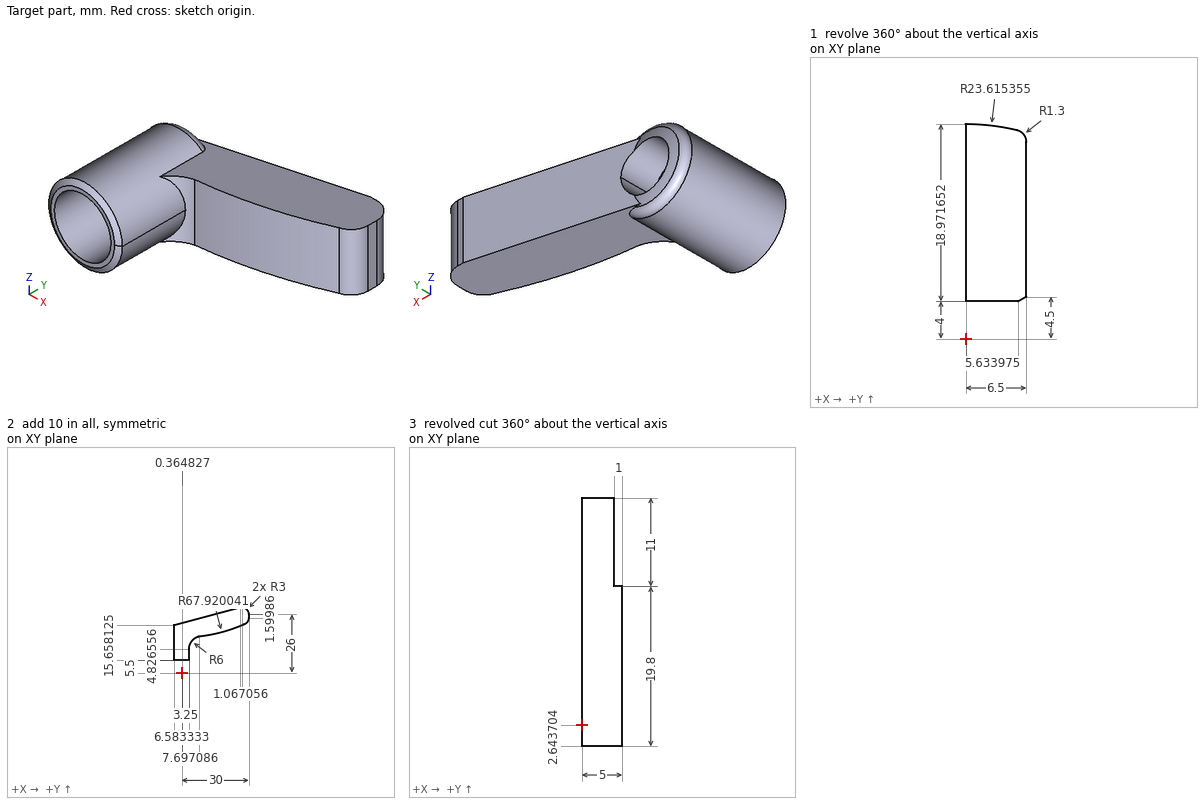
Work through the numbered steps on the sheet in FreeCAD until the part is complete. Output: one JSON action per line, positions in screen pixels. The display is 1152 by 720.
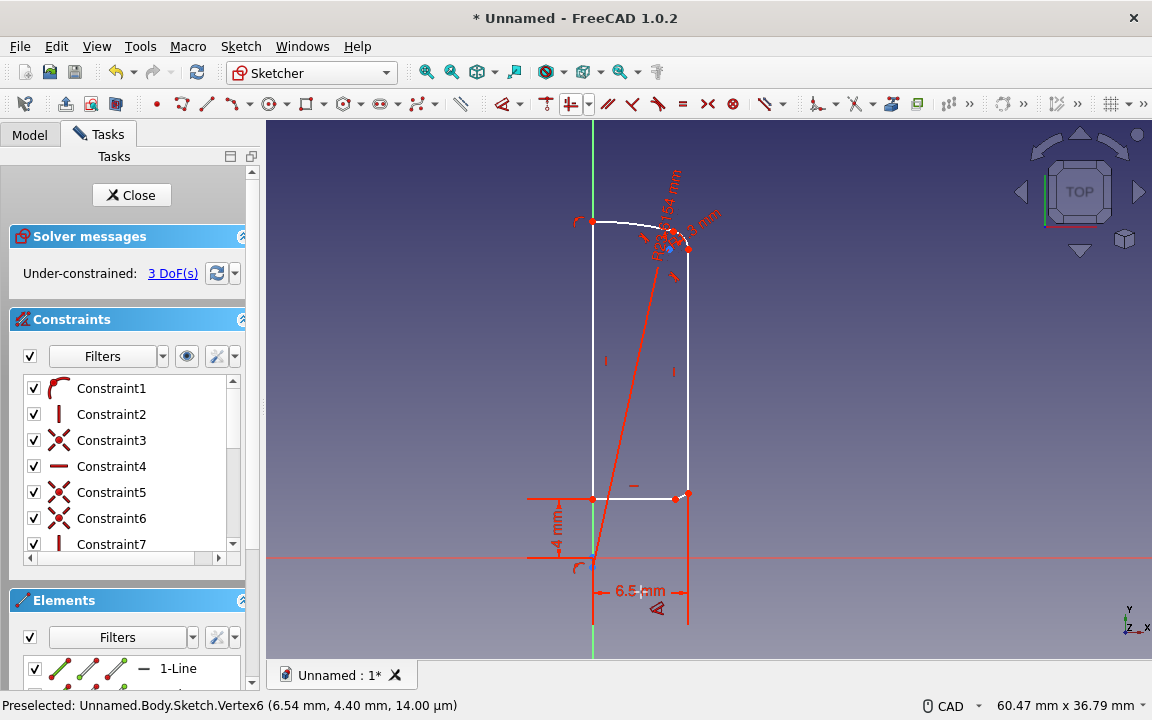
{"action": "left_click", "coordinate": [688, 494]}
{"action": "left_click", "coordinate": [722, 526]}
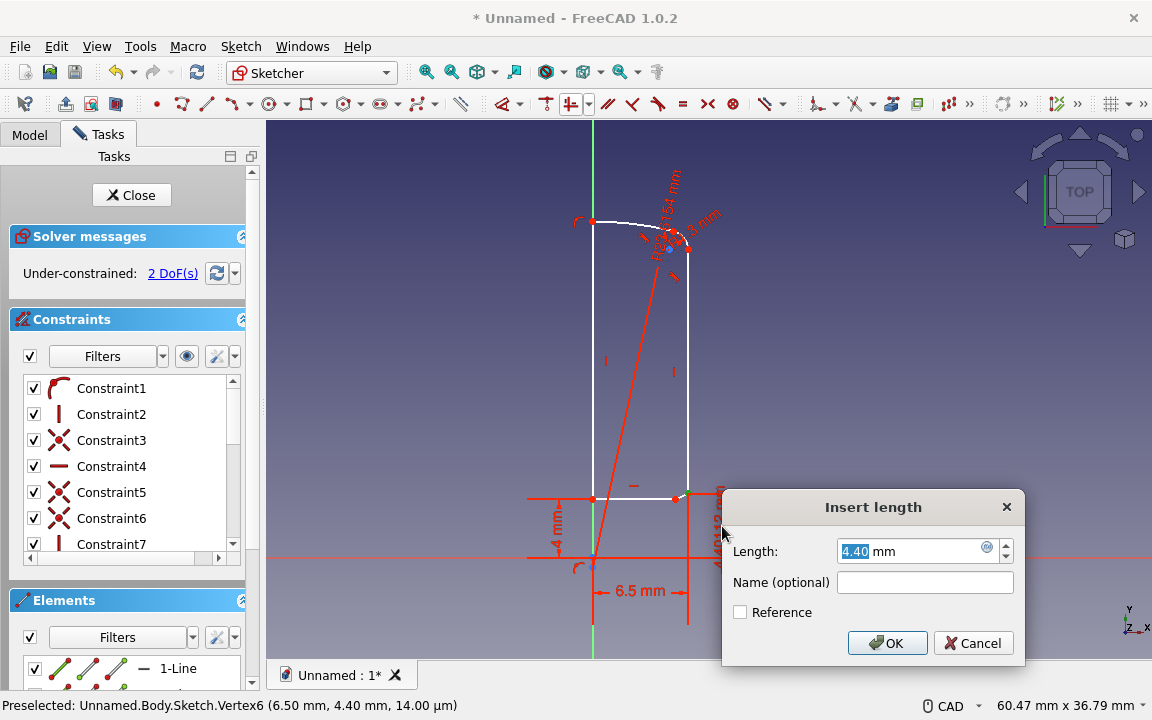
{"action": "type", "text": "4.5"}
{"action": "key", "text": "Return"}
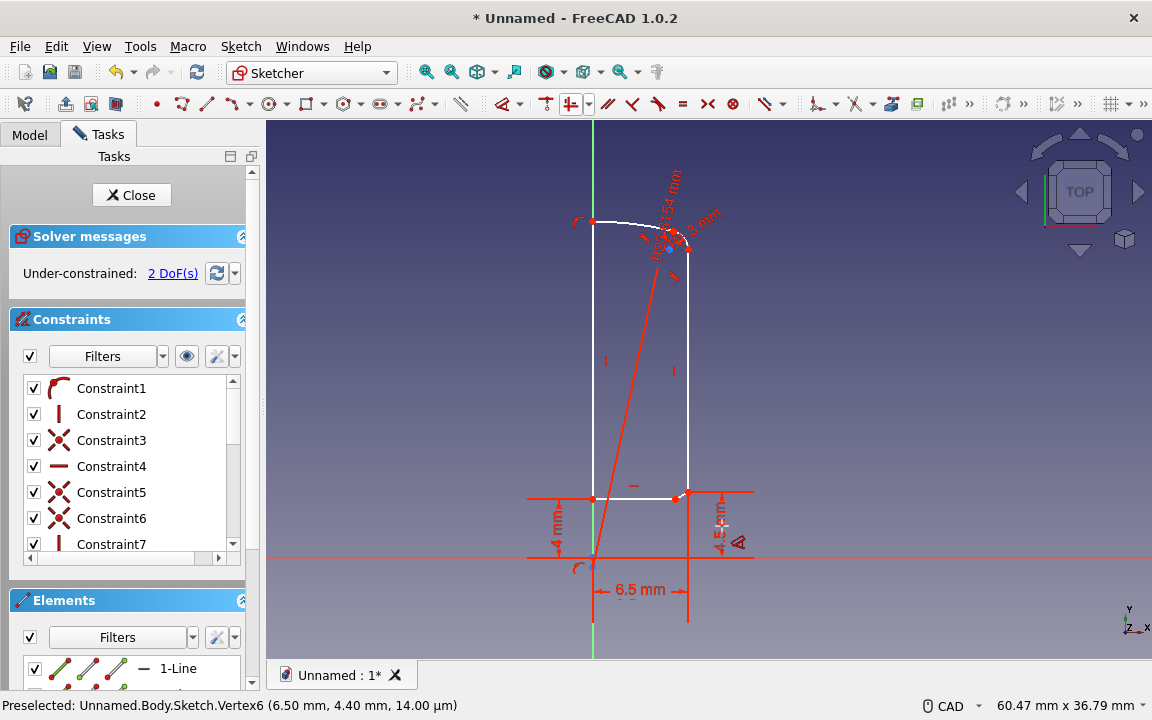
{"action": "left_click", "coordinate": [618, 499]}
{"action": "left_click", "coordinate": [634, 533]}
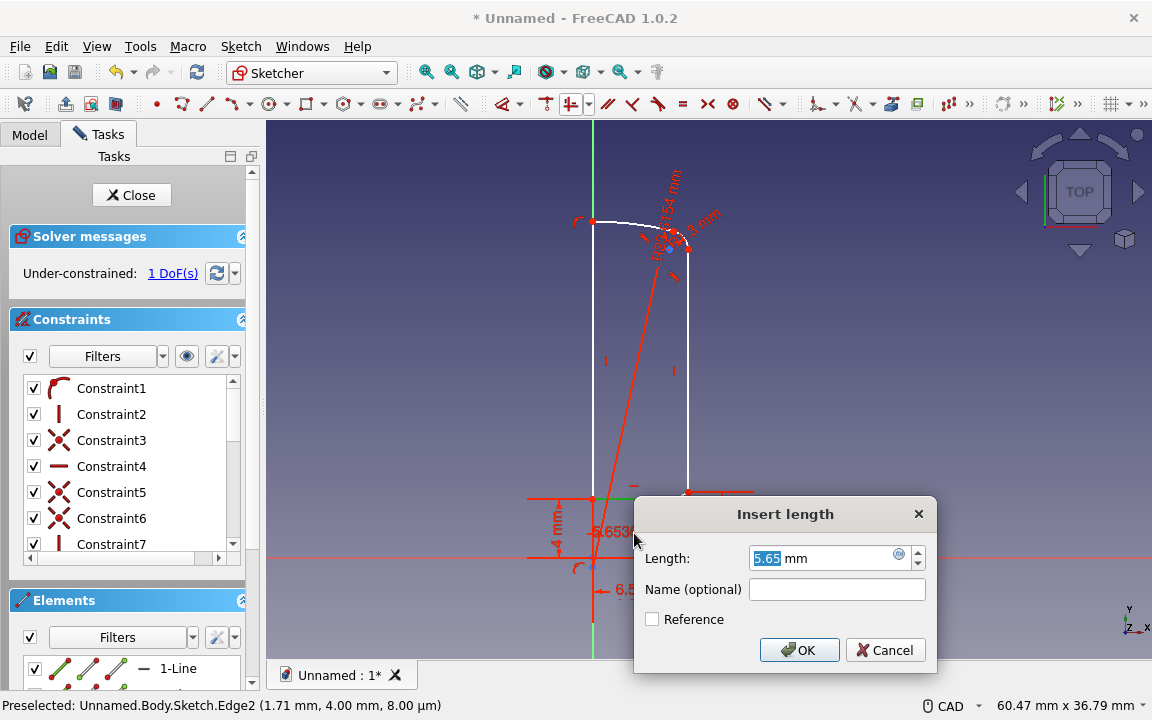
{"action": "type", "text": "5.633975"}
{"action": "key", "text": "Return"}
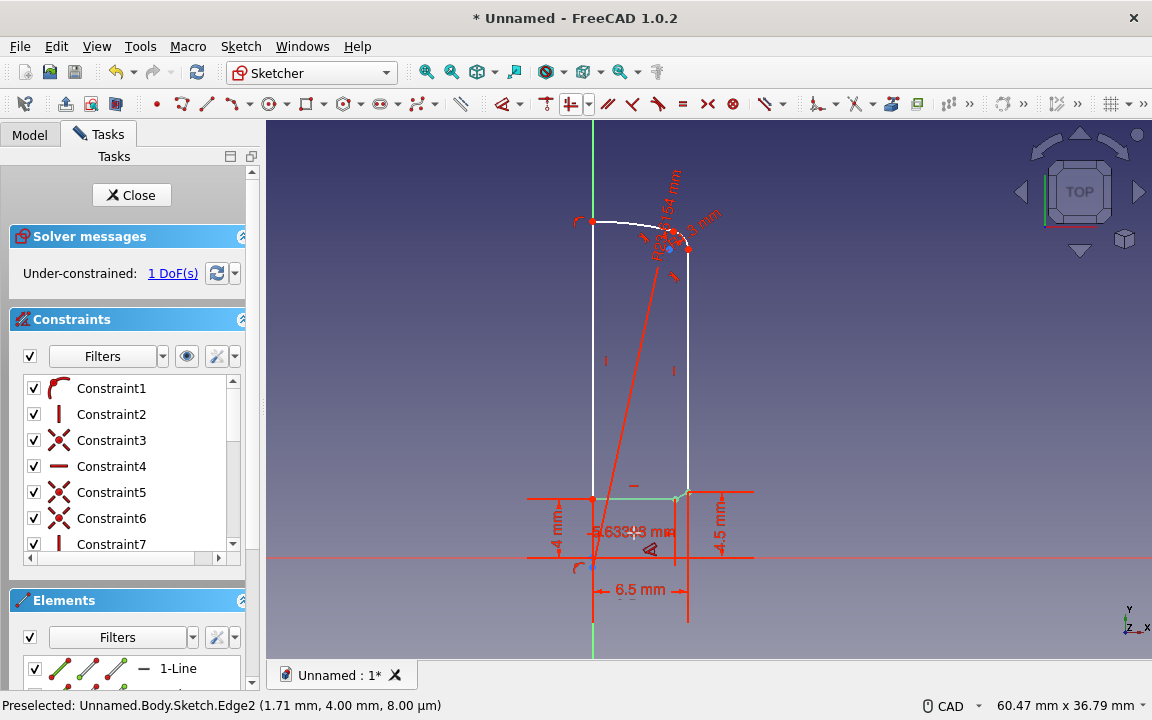
{"action": "left_click", "coordinate": [593, 305]}
{"action": "left_click", "coordinate": [559, 361]}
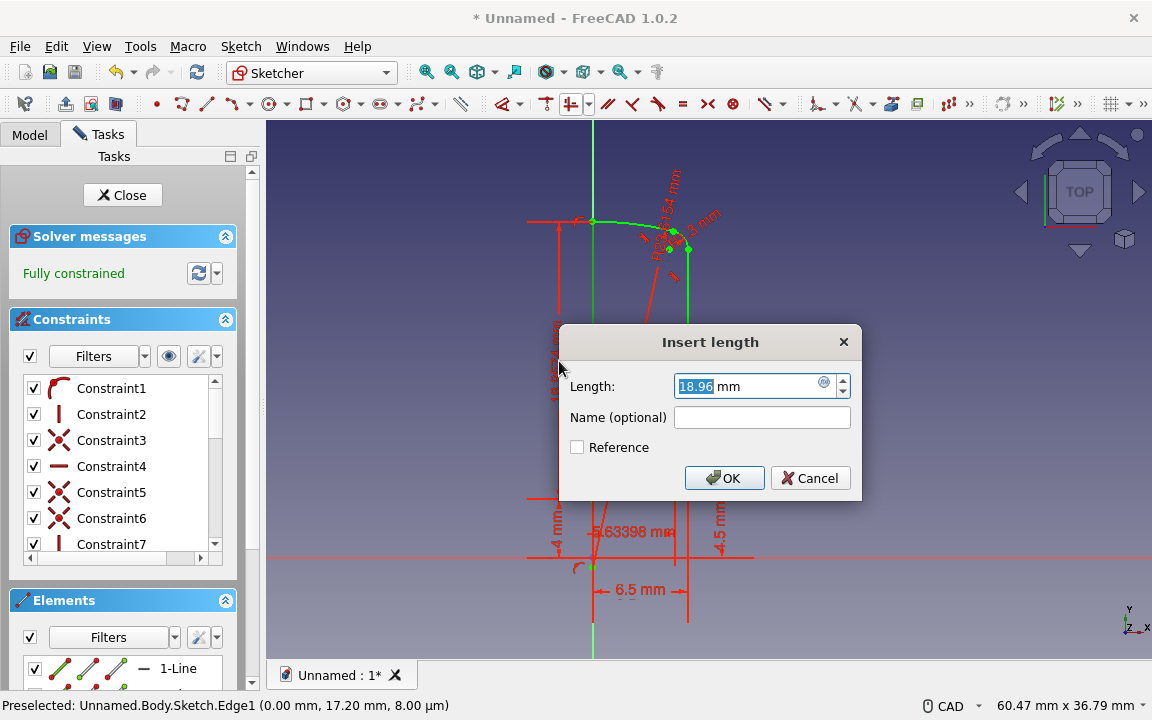
{"action": "type", "text": "18.971652"}
{"action": "key", "text": "Return"}
{"action": "key", "text": "Escape"}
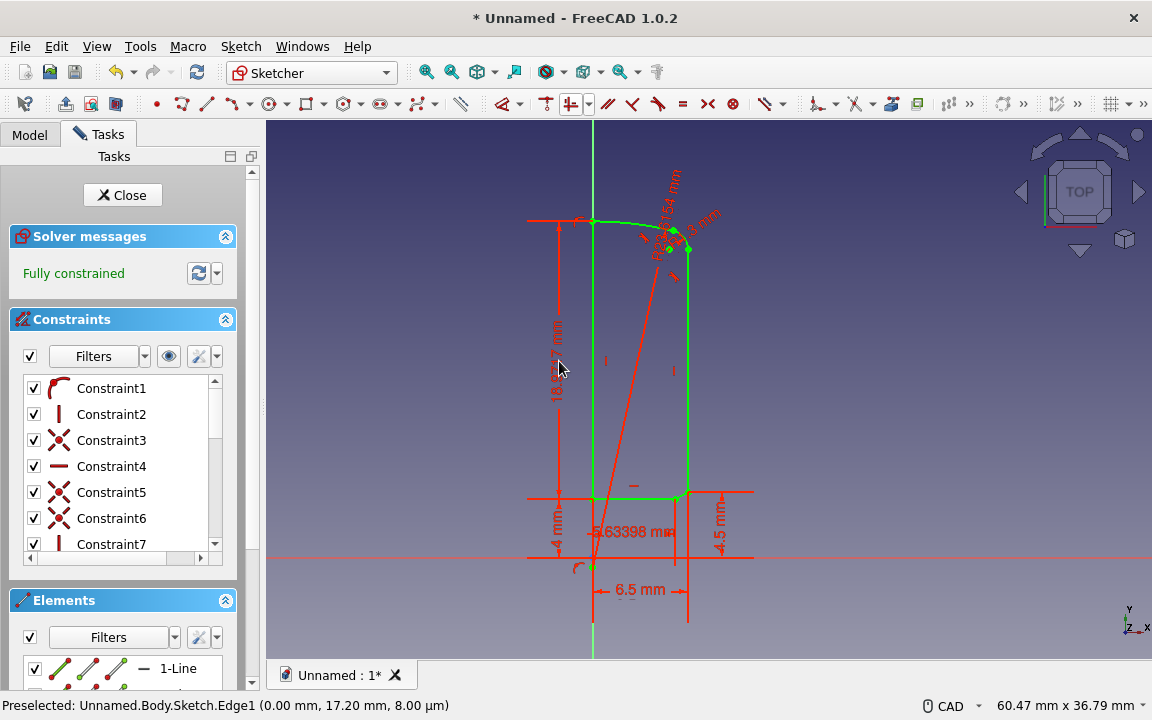
{"action": "left_click", "coordinate": [123, 195]}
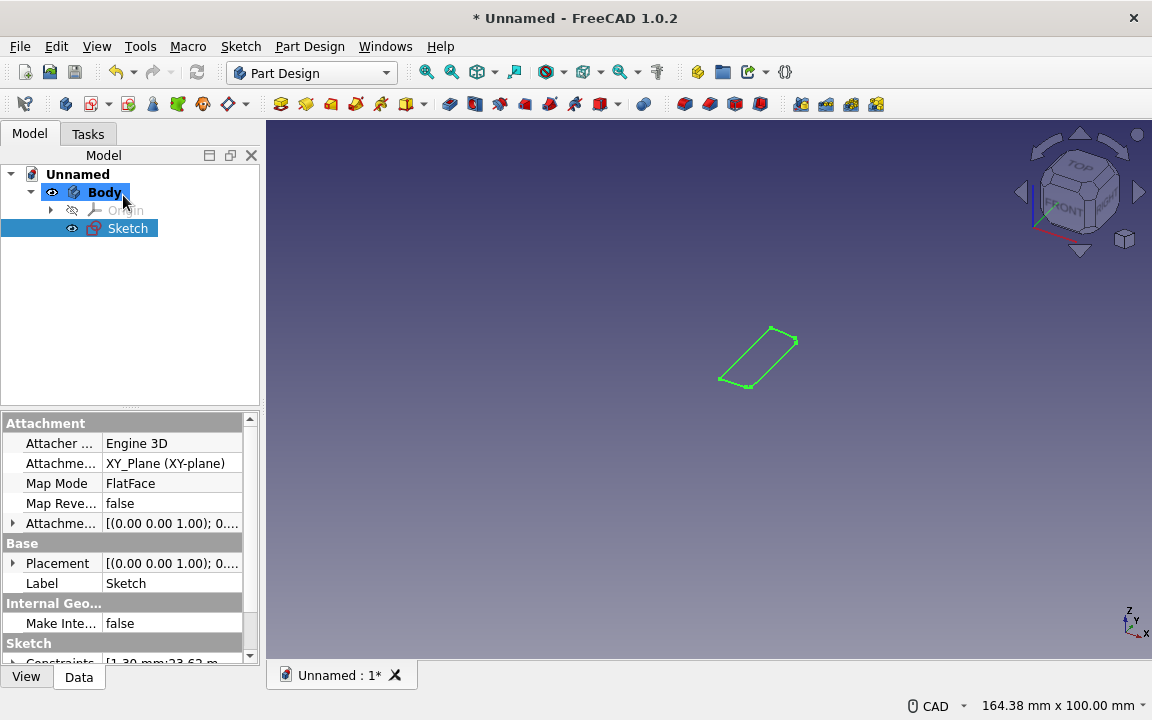
{"action": "left_click", "coordinate": [306, 104]}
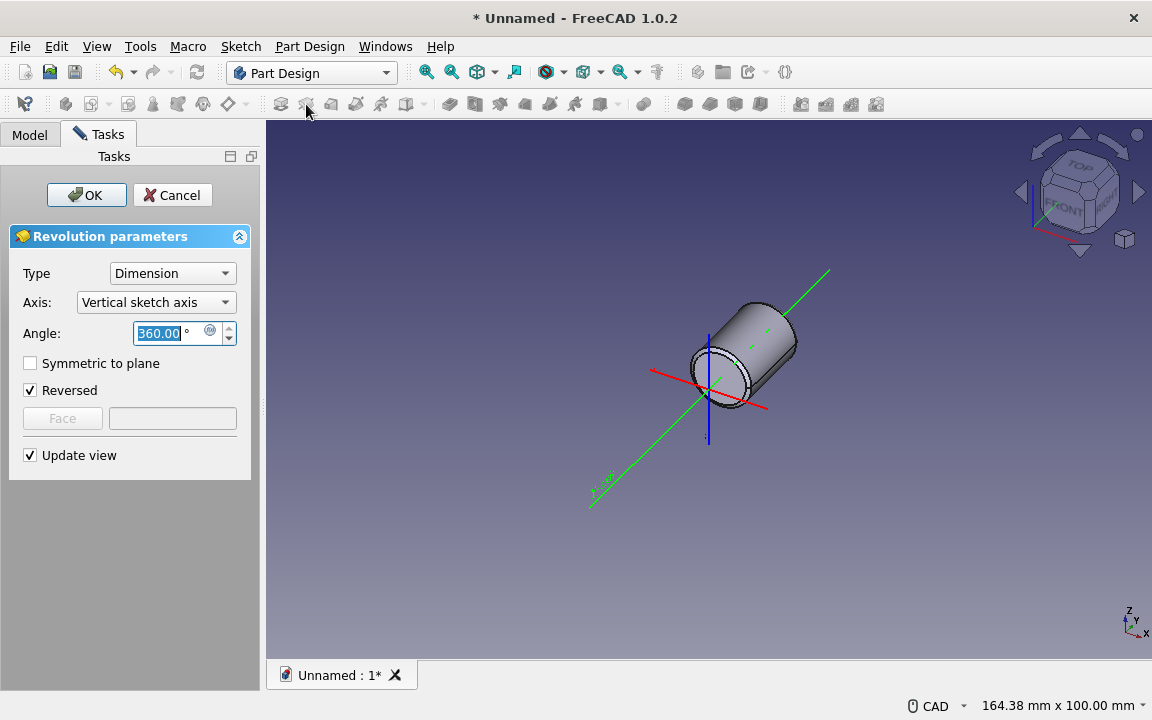
{"action": "left_click", "coordinate": [87, 195]}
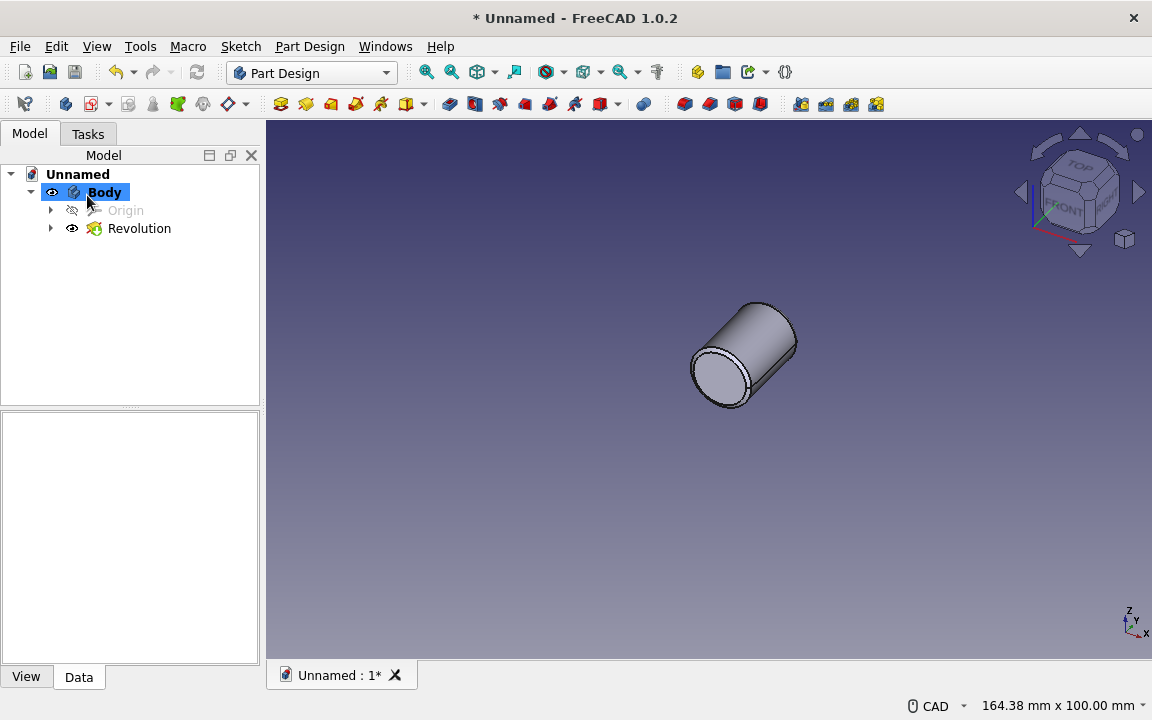
{"action": "key", "text": "v f"}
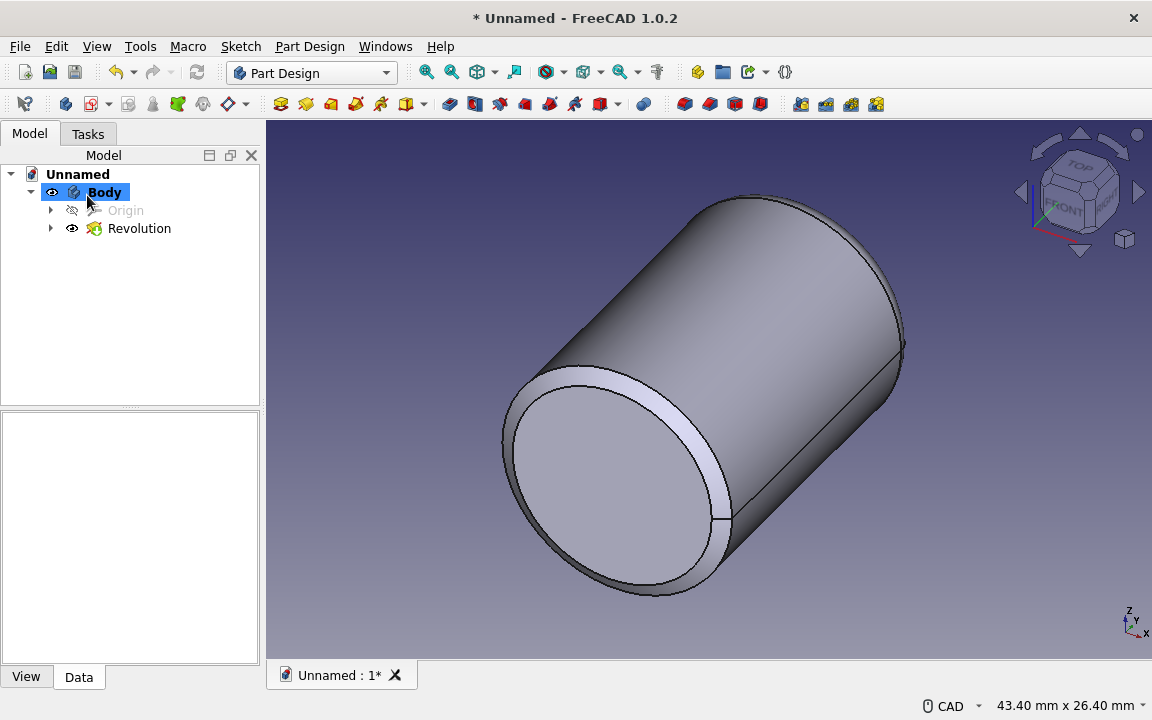
{"action": "left_click", "coordinate": [90, 104]}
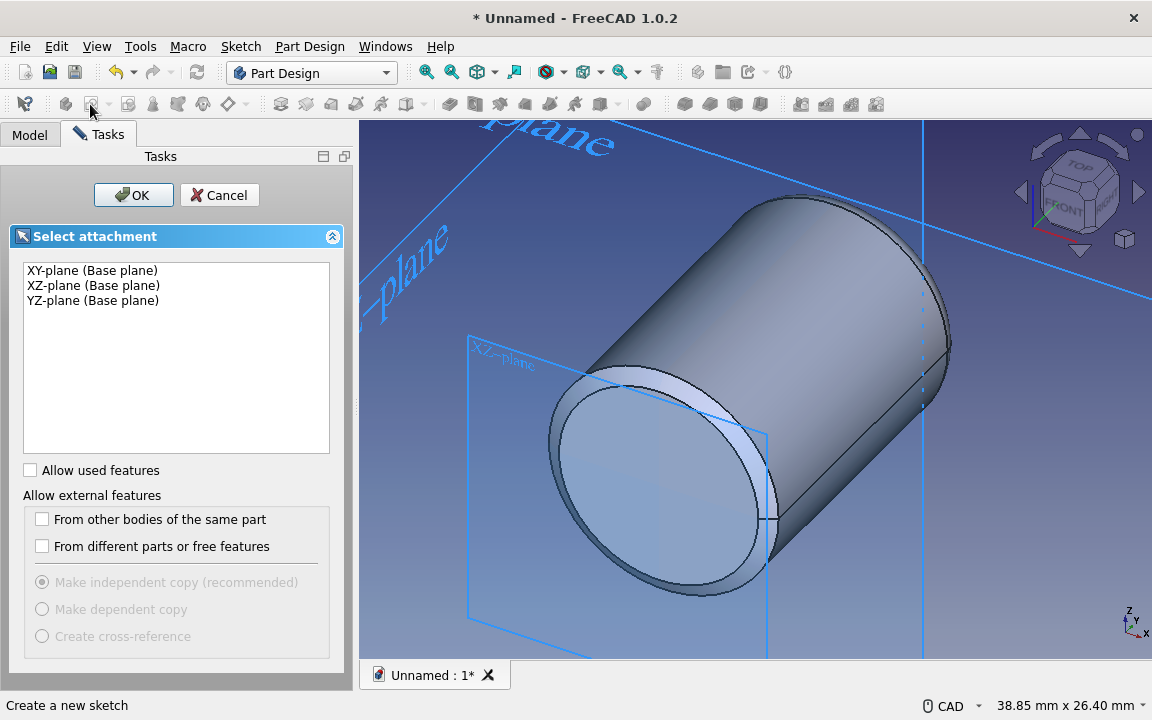
{"action": "left_click", "coordinate": [84, 270]}